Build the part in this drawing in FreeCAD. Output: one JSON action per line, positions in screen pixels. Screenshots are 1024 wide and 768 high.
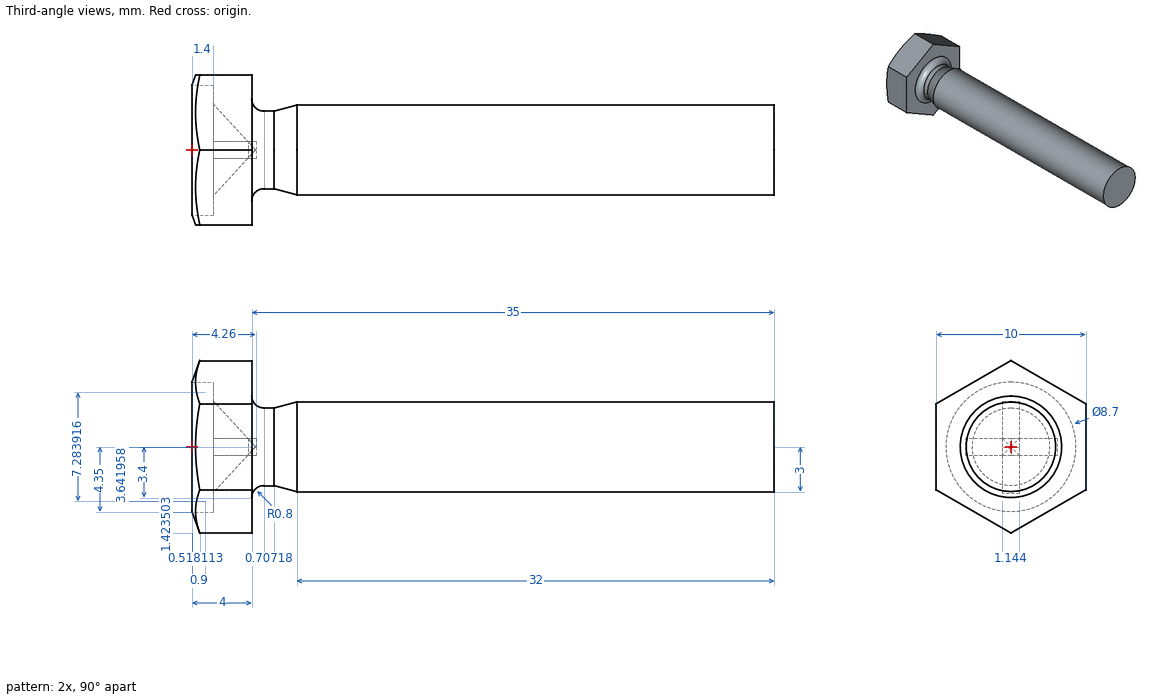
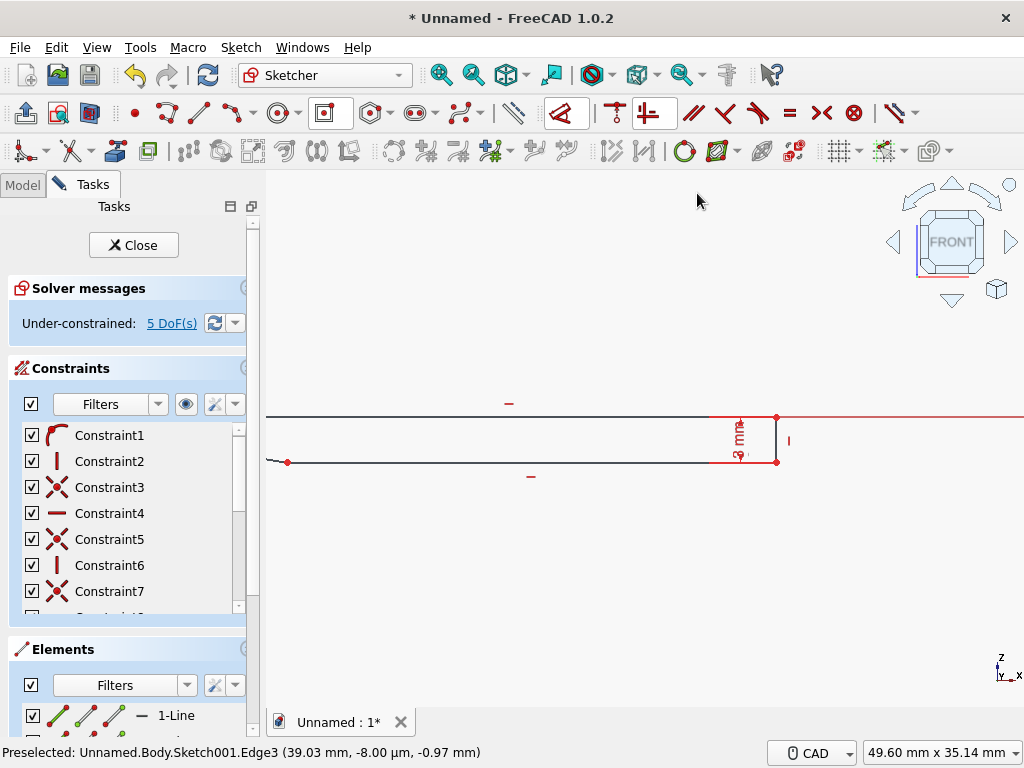
{"action": "left_click", "coordinate": [402, 417]}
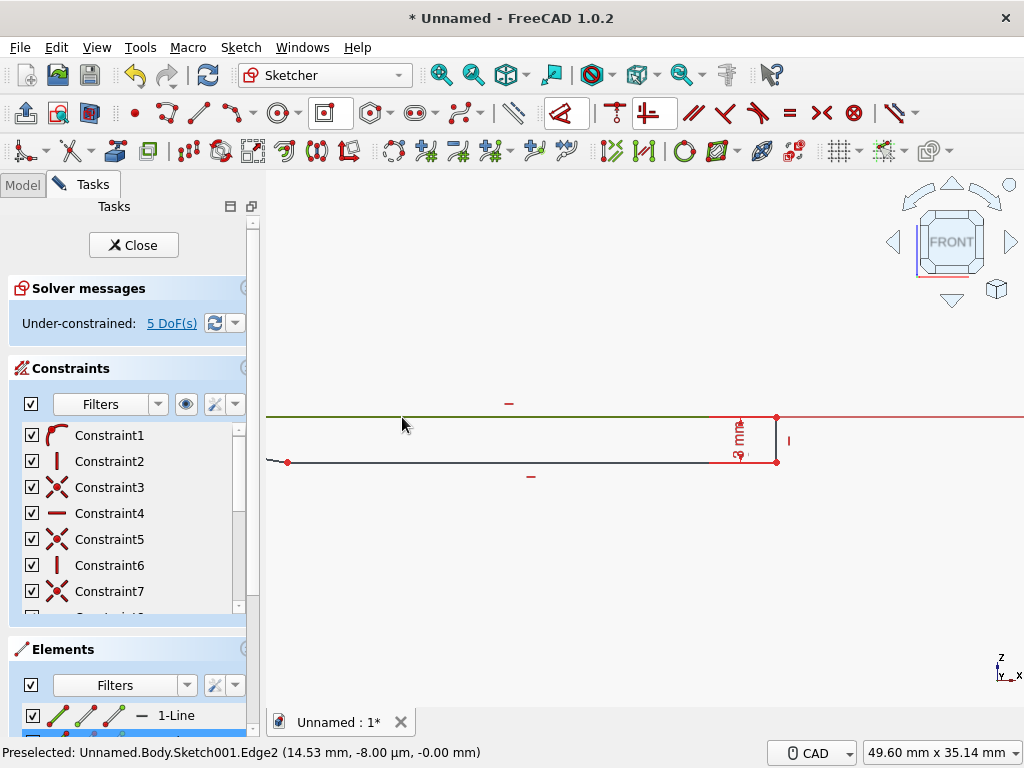
{"action": "key", "text": "l"}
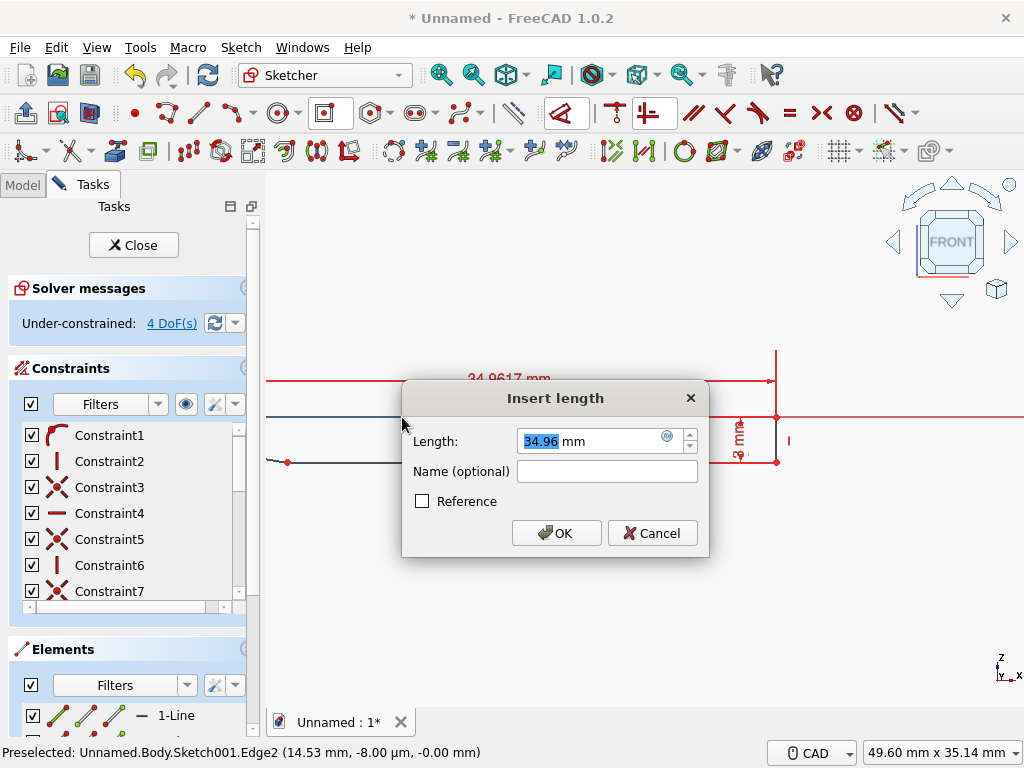
{"action": "type", "text": "35"}
{"action": "key", "text": "Return"}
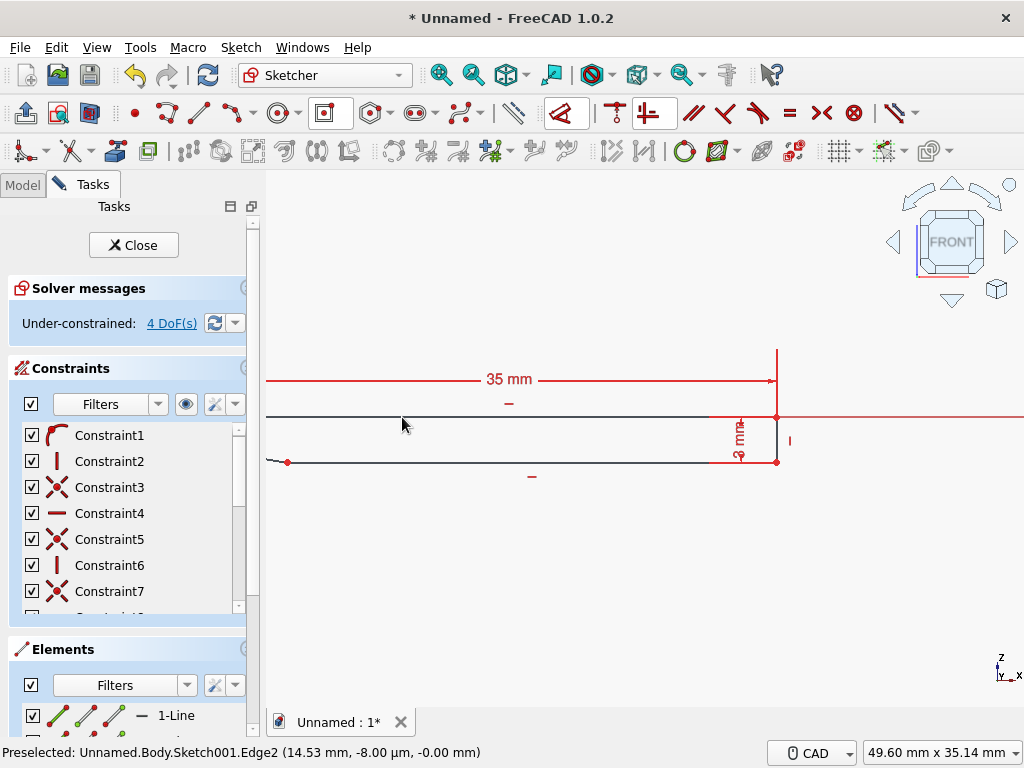
{"action": "left_click", "coordinate": [630, 463]}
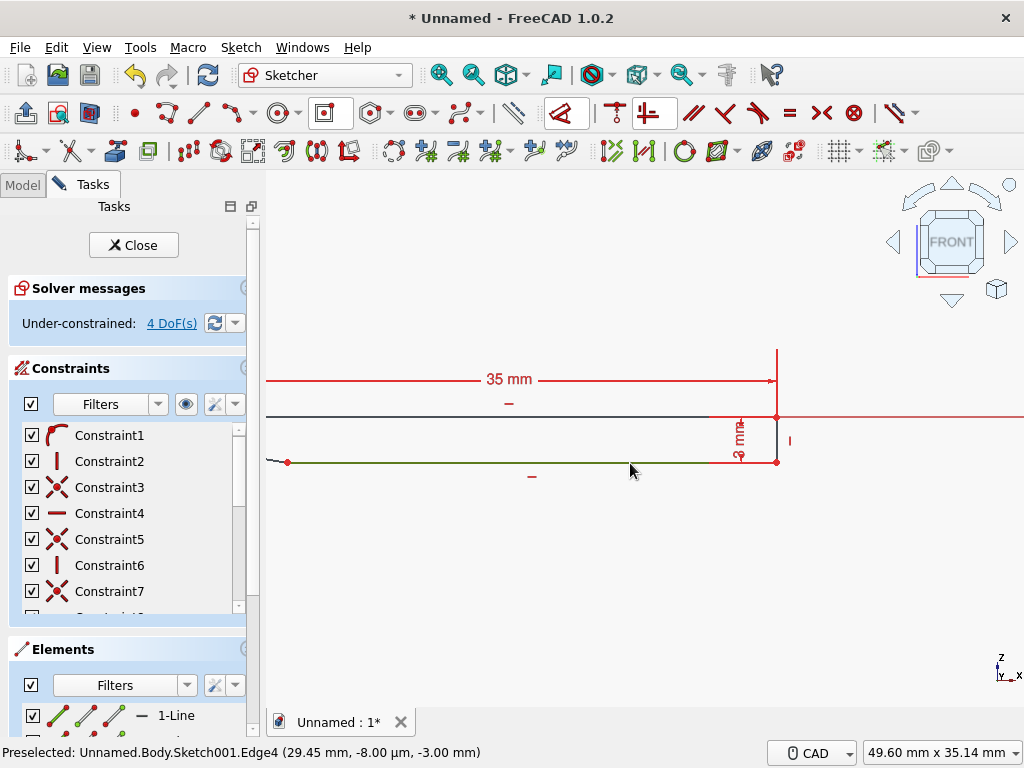
{"action": "key", "text": "l"}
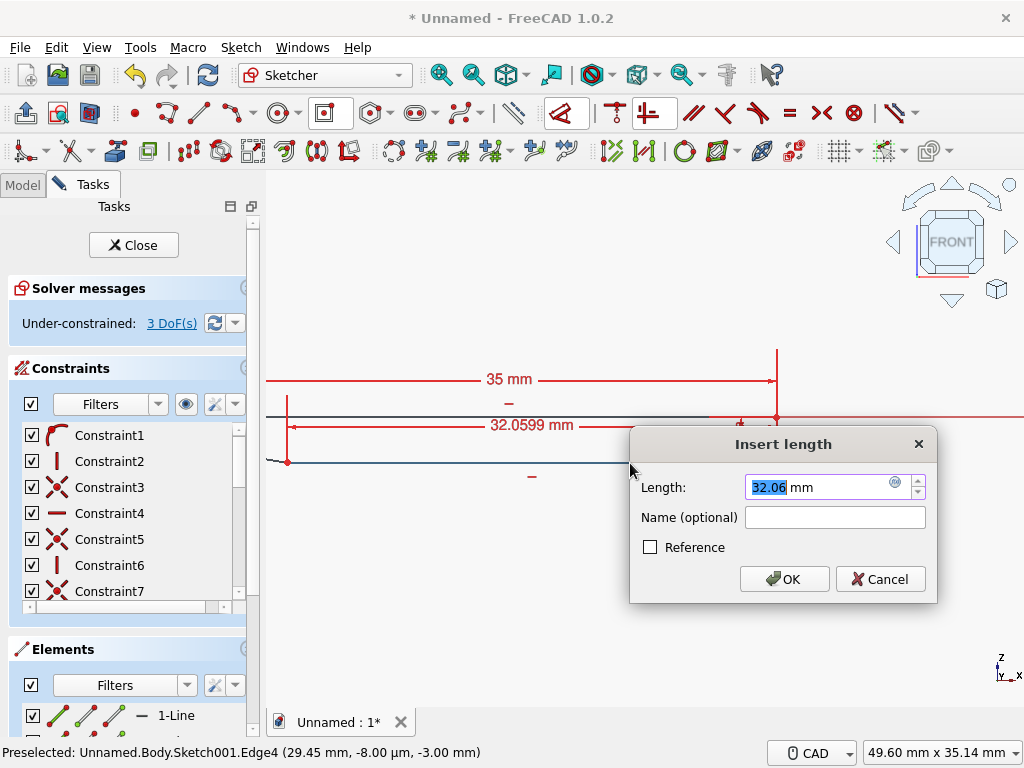
{"action": "type", "text": "32"}
{"action": "key", "text": "Return"}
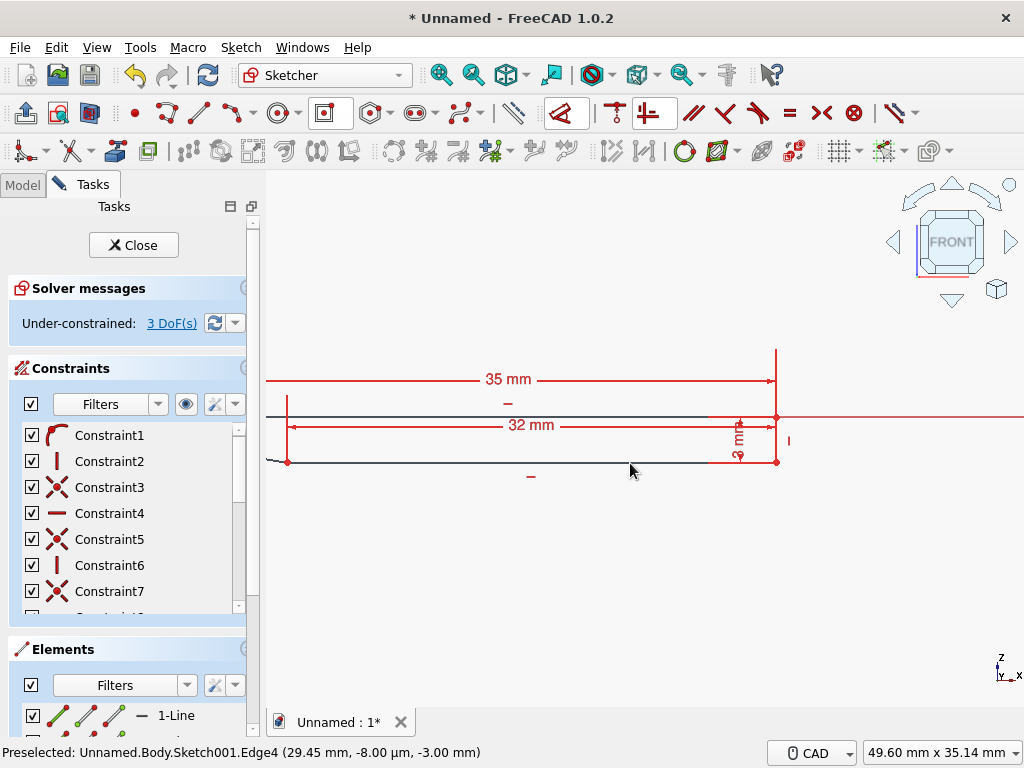
{"action": "scroll", "coordinate": [777, 429], "scroll_direction": "down", "scroll_amount": 2}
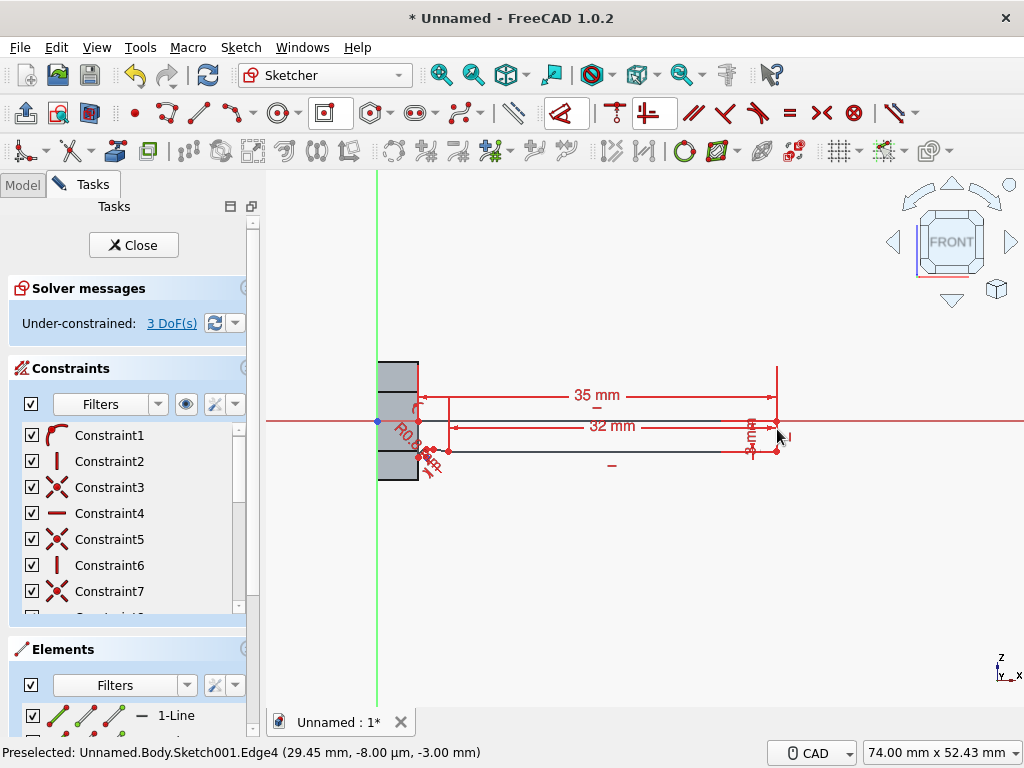
{"action": "scroll", "coordinate": [418, 457], "scroll_direction": "up", "scroll_amount": 2}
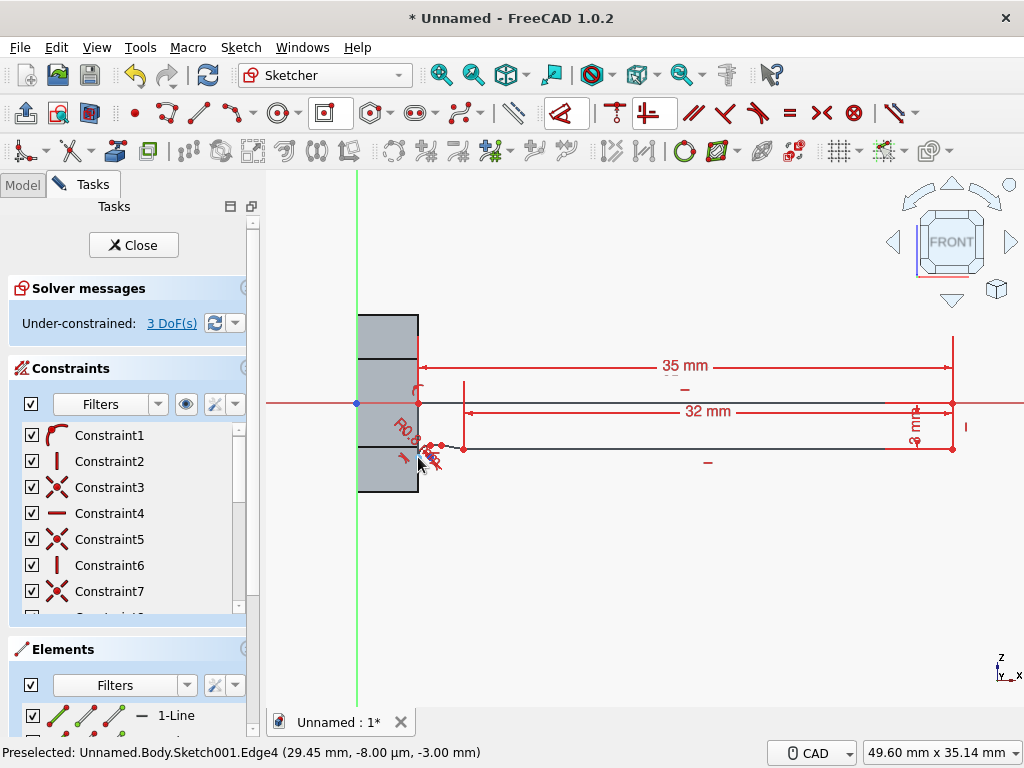
{"action": "left_click", "coordinate": [418, 457]}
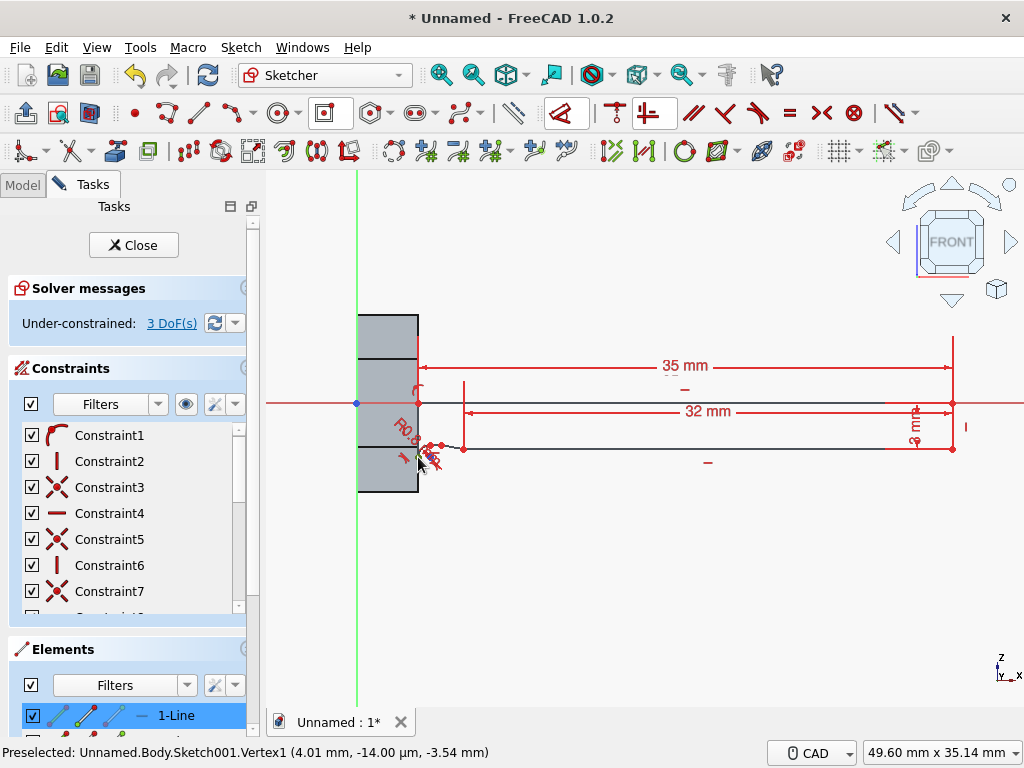
{"action": "left_click", "coordinate": [584, 114]}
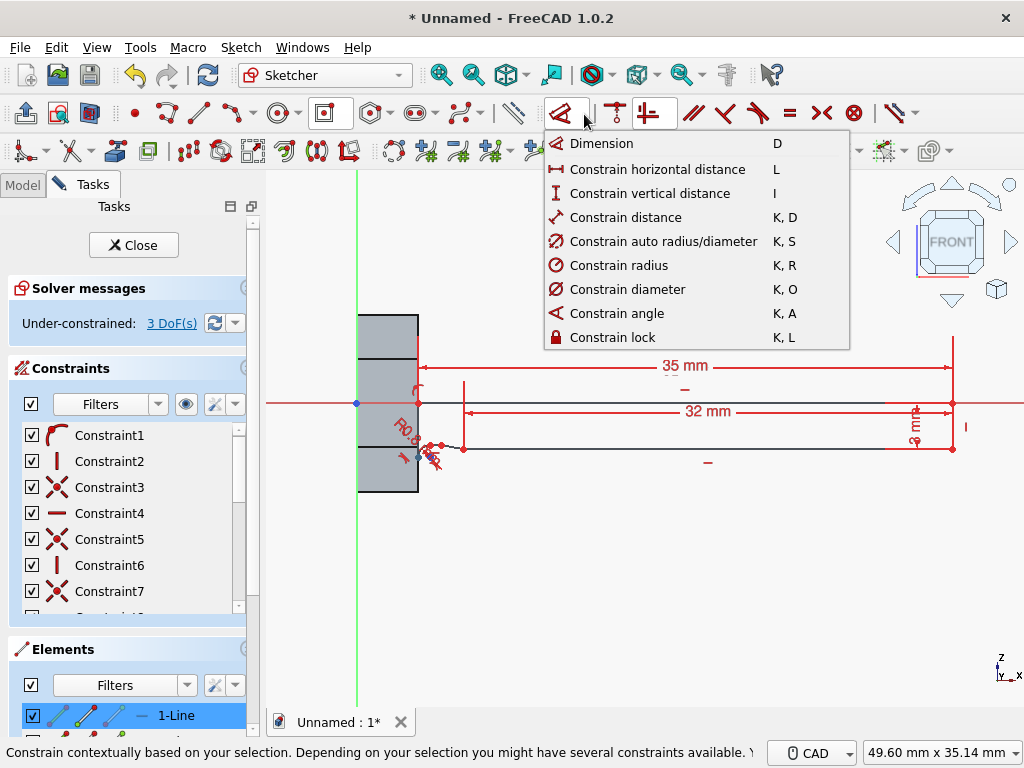
{"action": "left_click", "coordinate": [697, 169]}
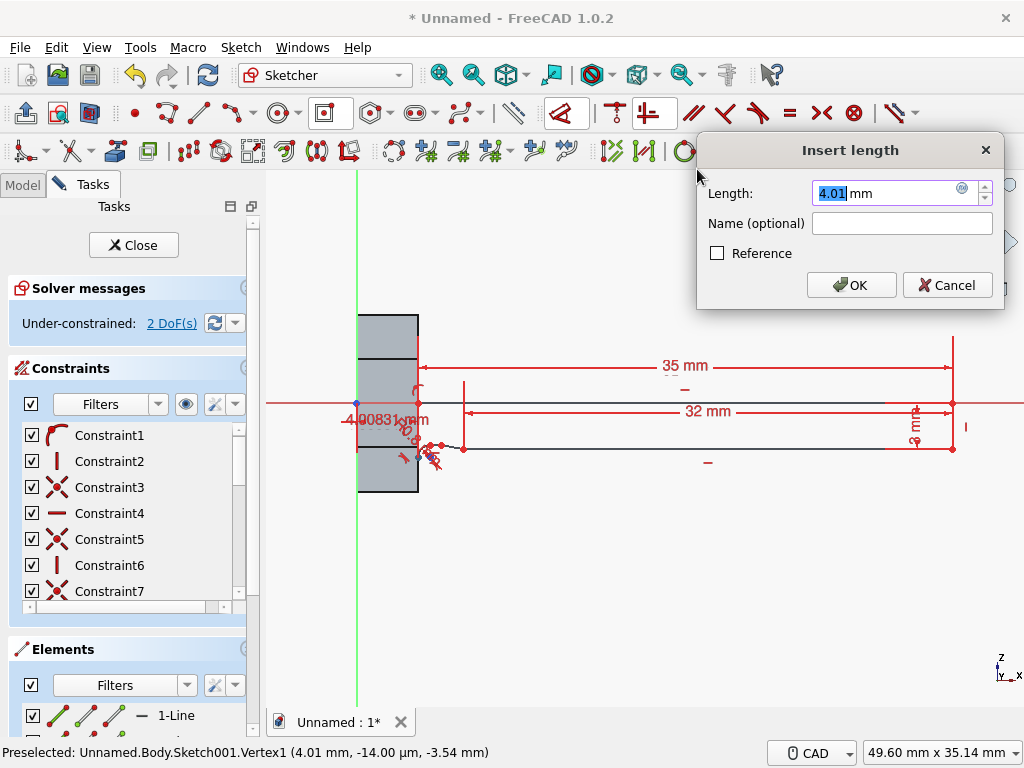
{"action": "type", "text": "4"}
{"action": "key", "text": "Return"}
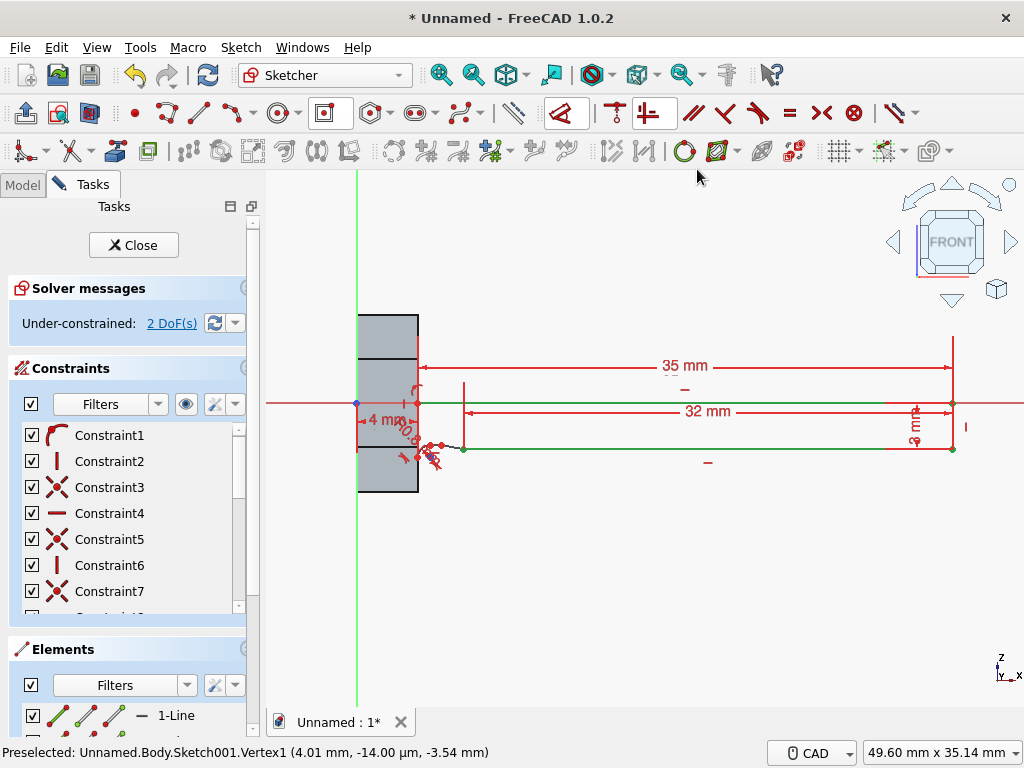
{"action": "left_click", "coordinate": [418, 420]}